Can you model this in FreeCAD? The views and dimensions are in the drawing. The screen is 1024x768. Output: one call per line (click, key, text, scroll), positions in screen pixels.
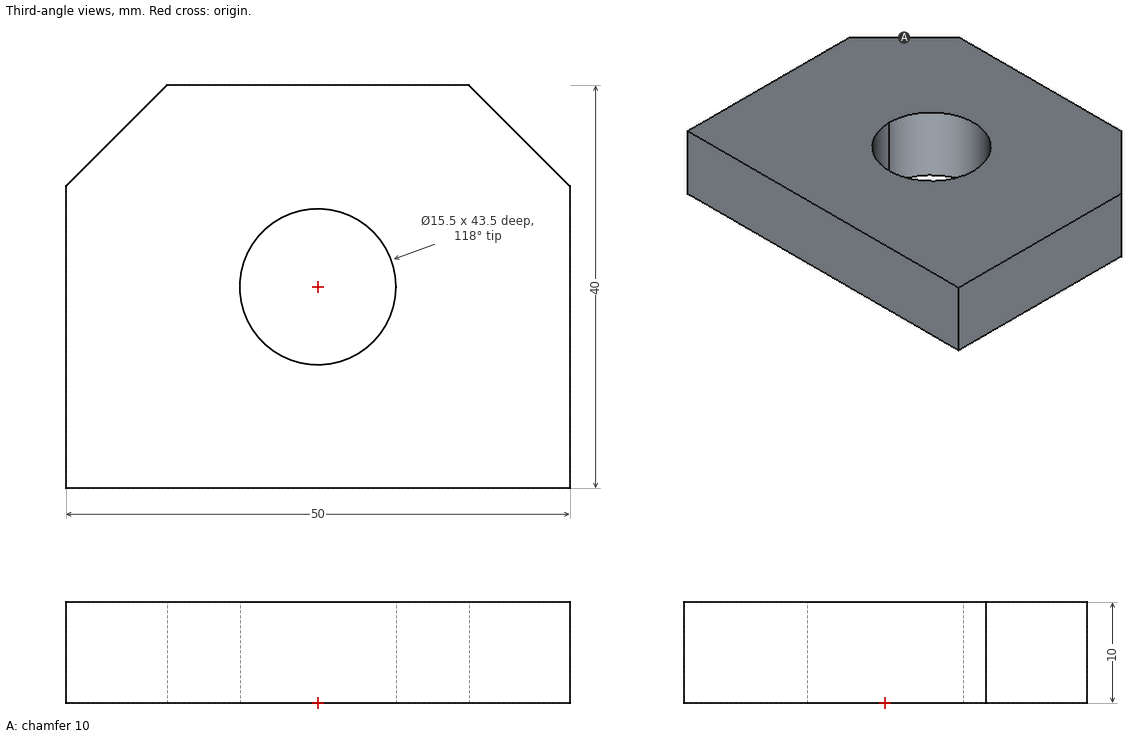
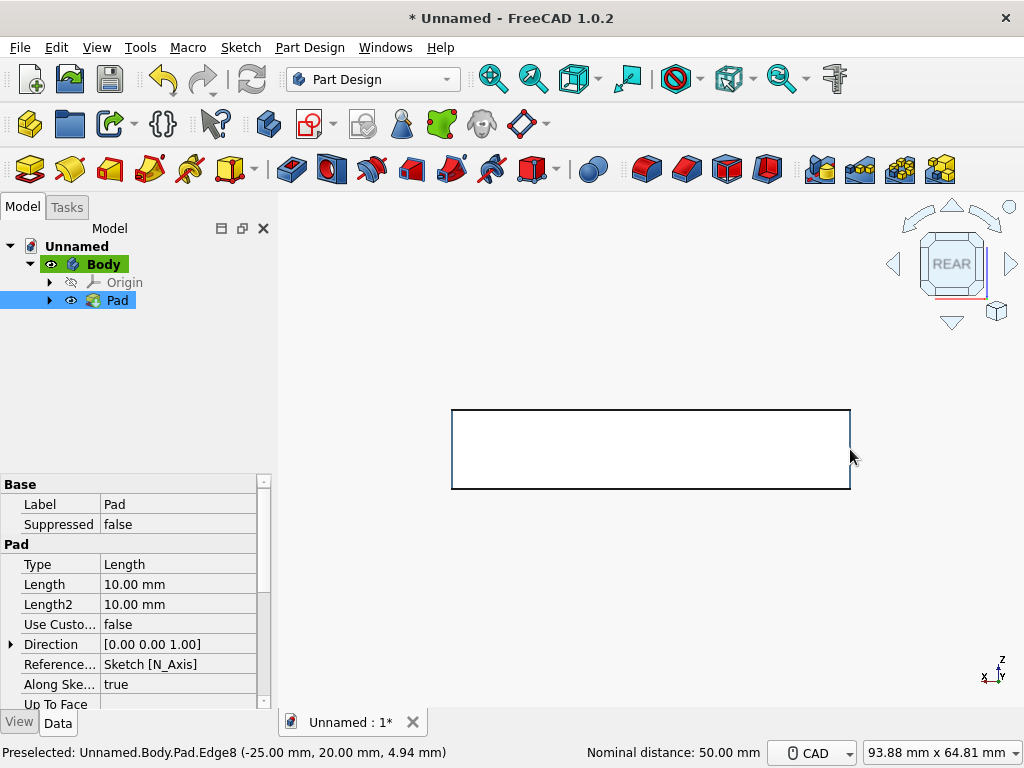
click(688, 170)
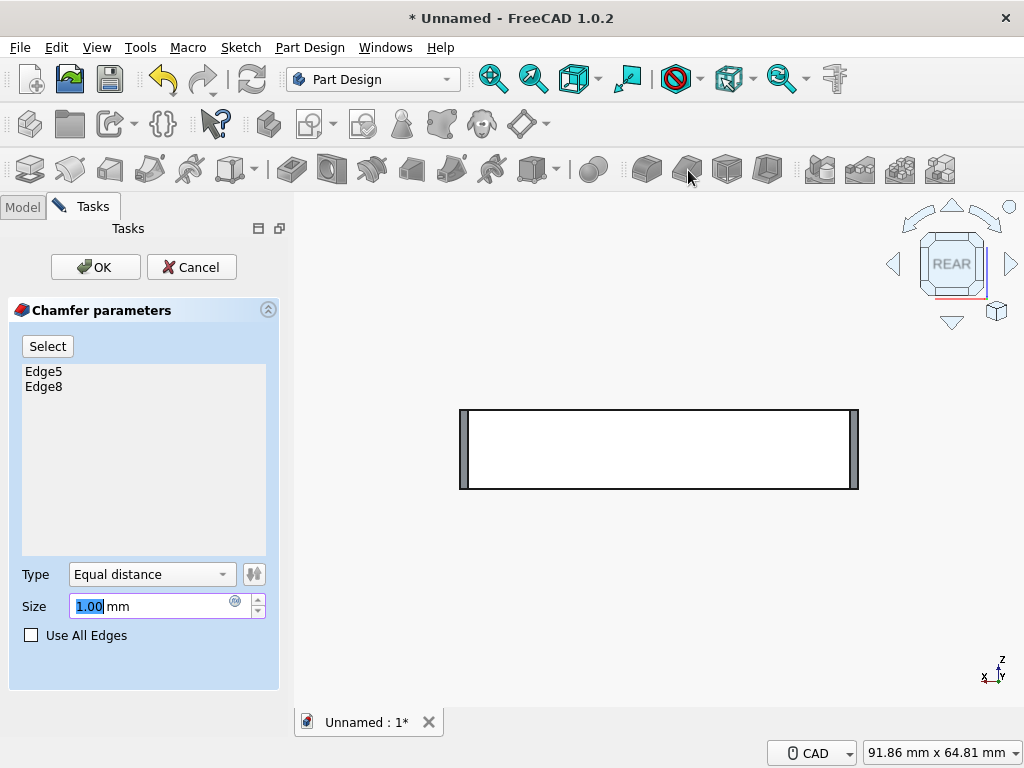
text(10)
key(Tab)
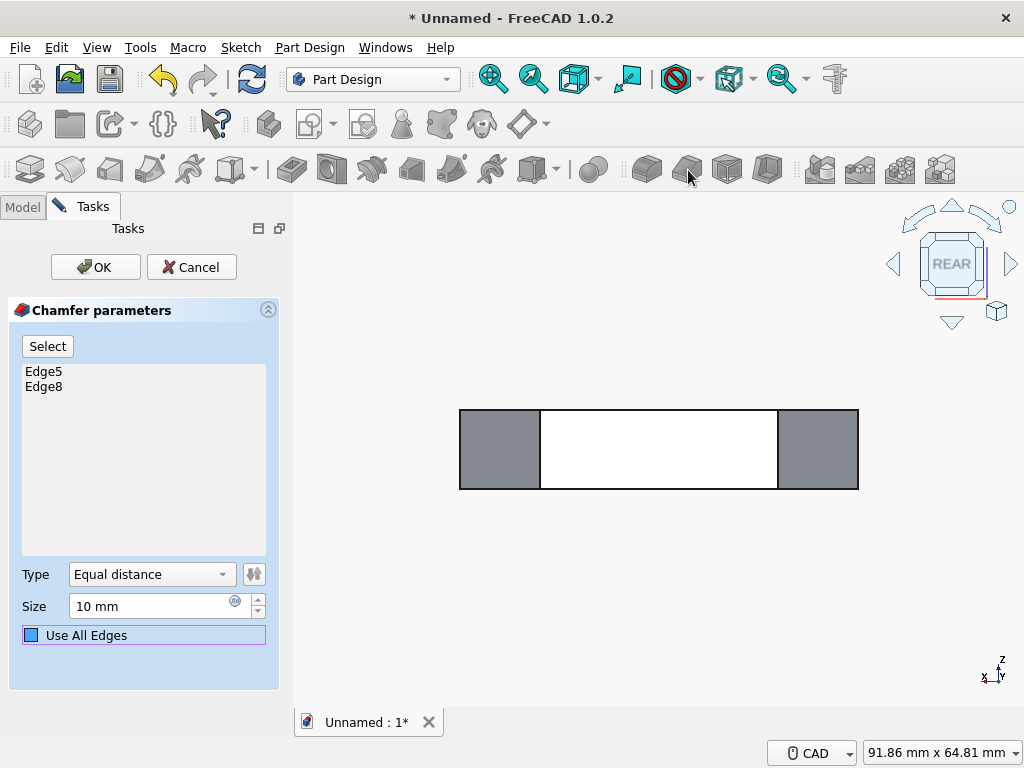
click(96, 267)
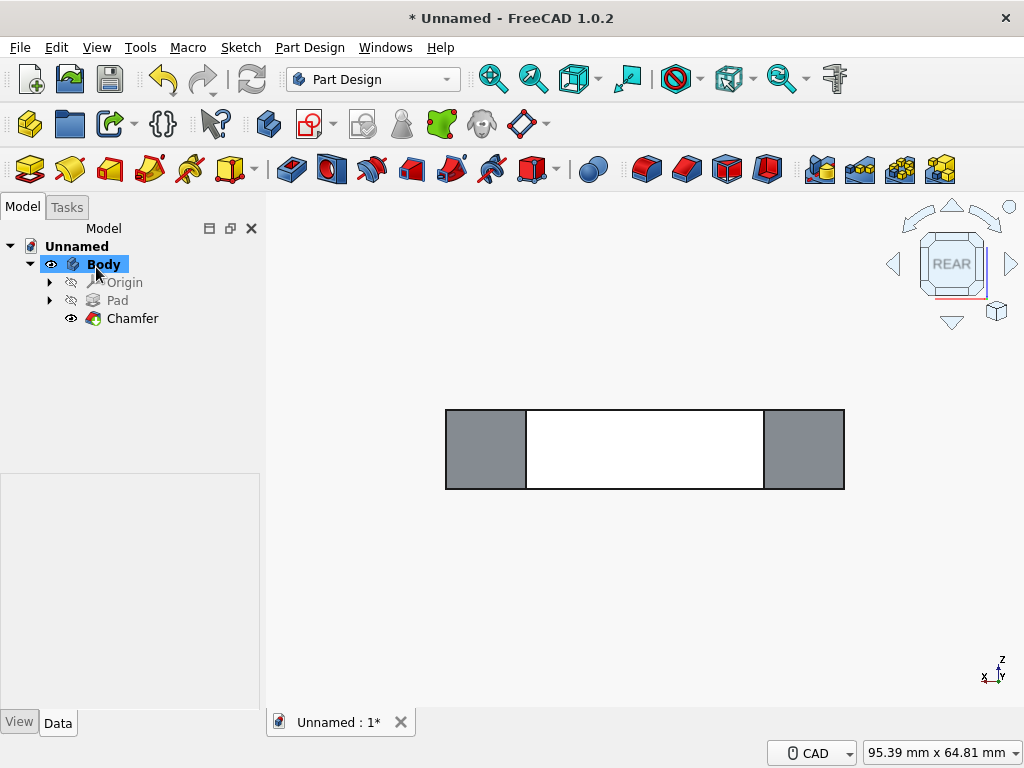
key(5)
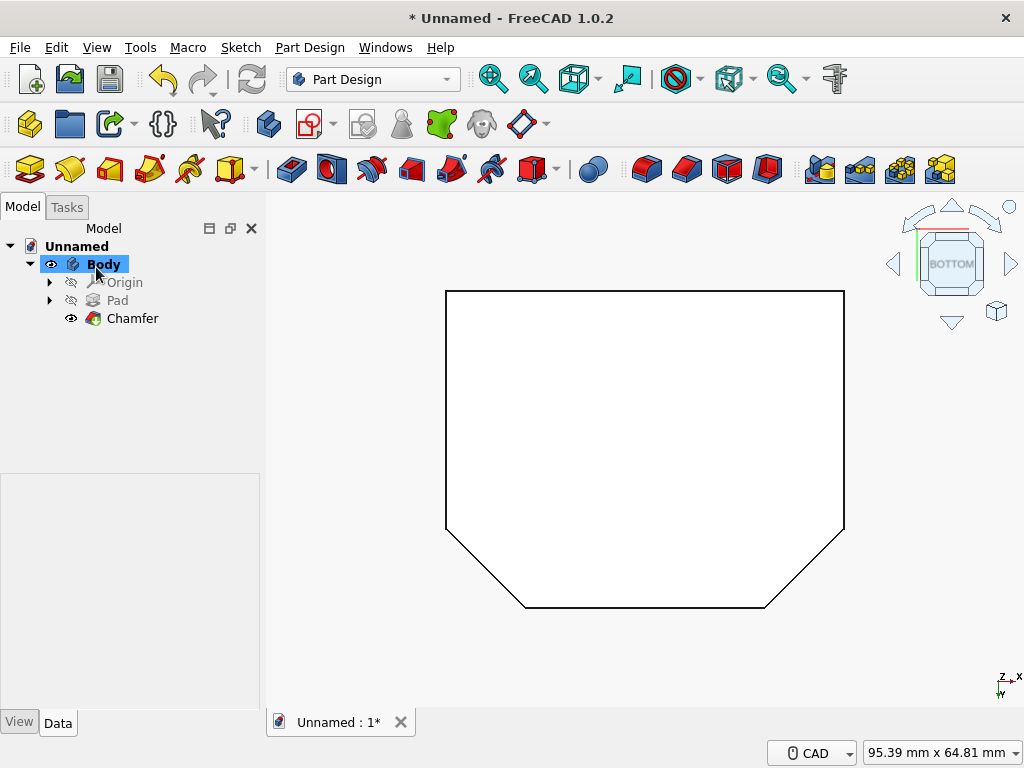
click(645, 448)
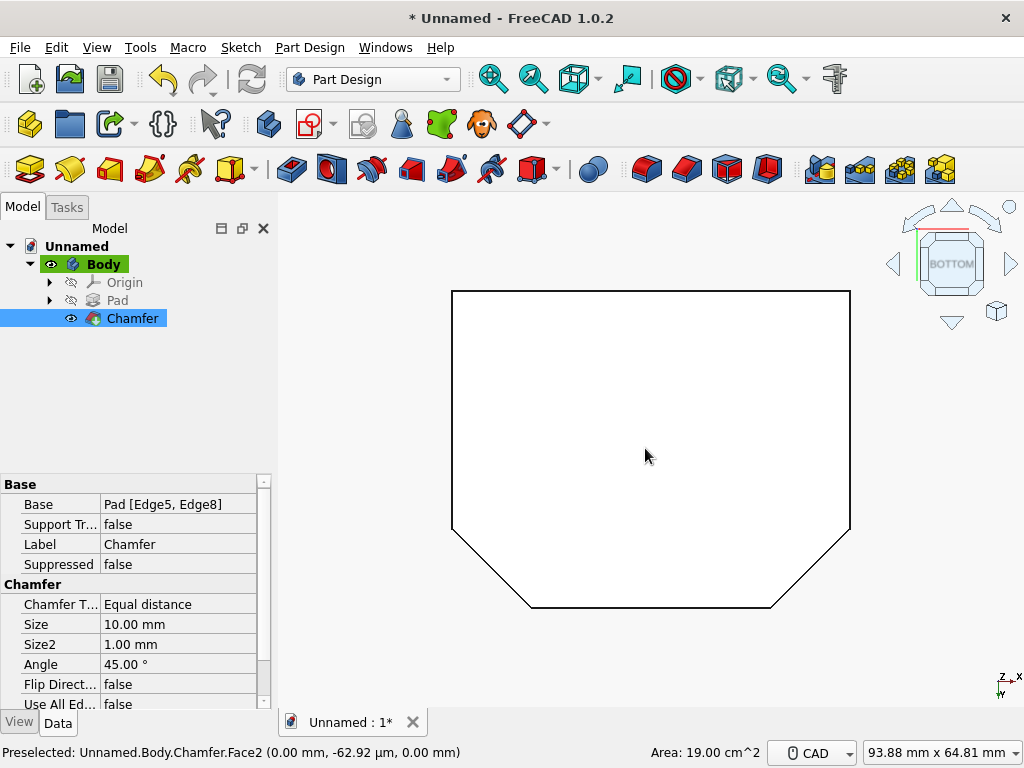
click(310, 124)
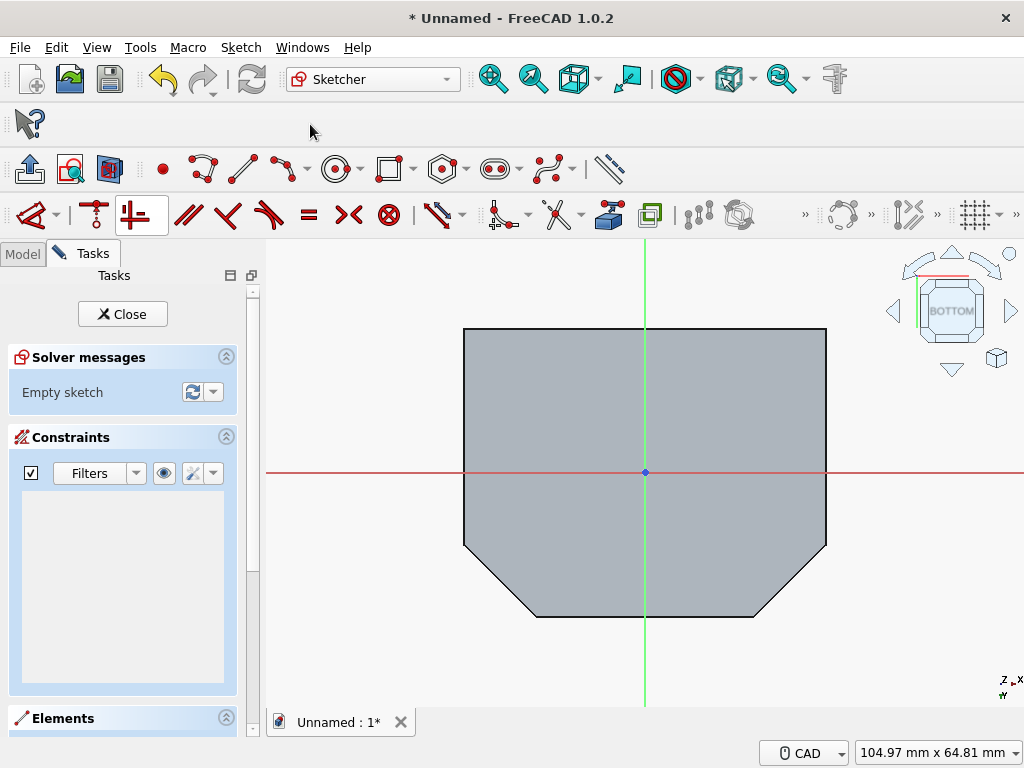
scroll(685, 473, up, 5)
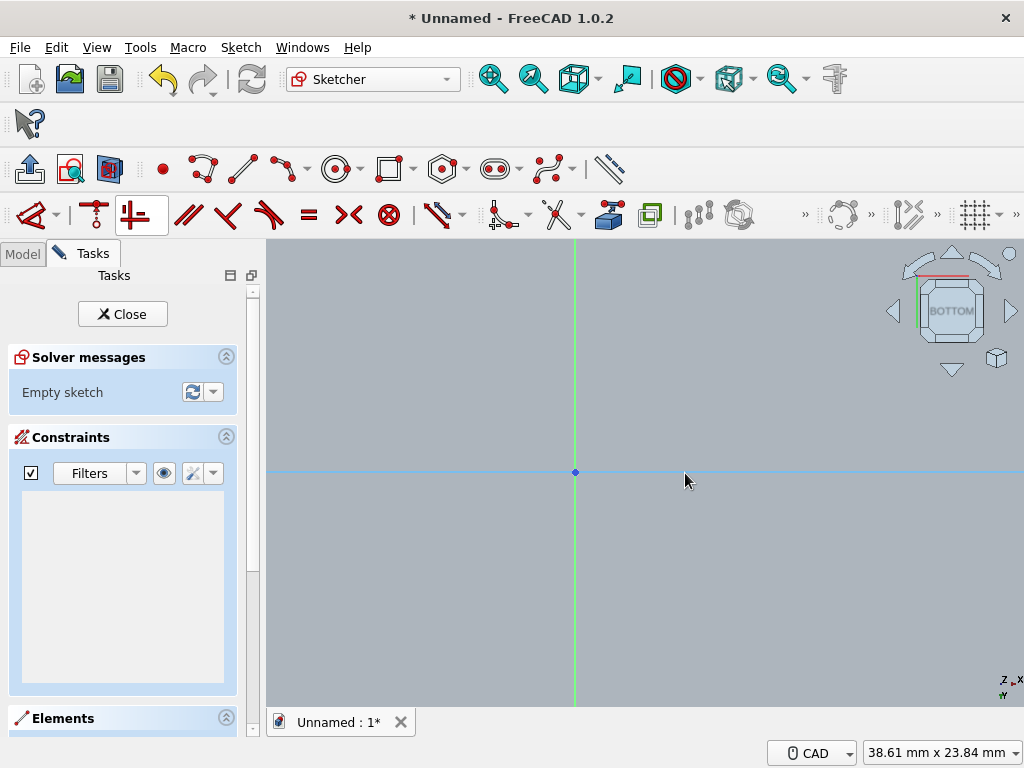
key(g)
key(c)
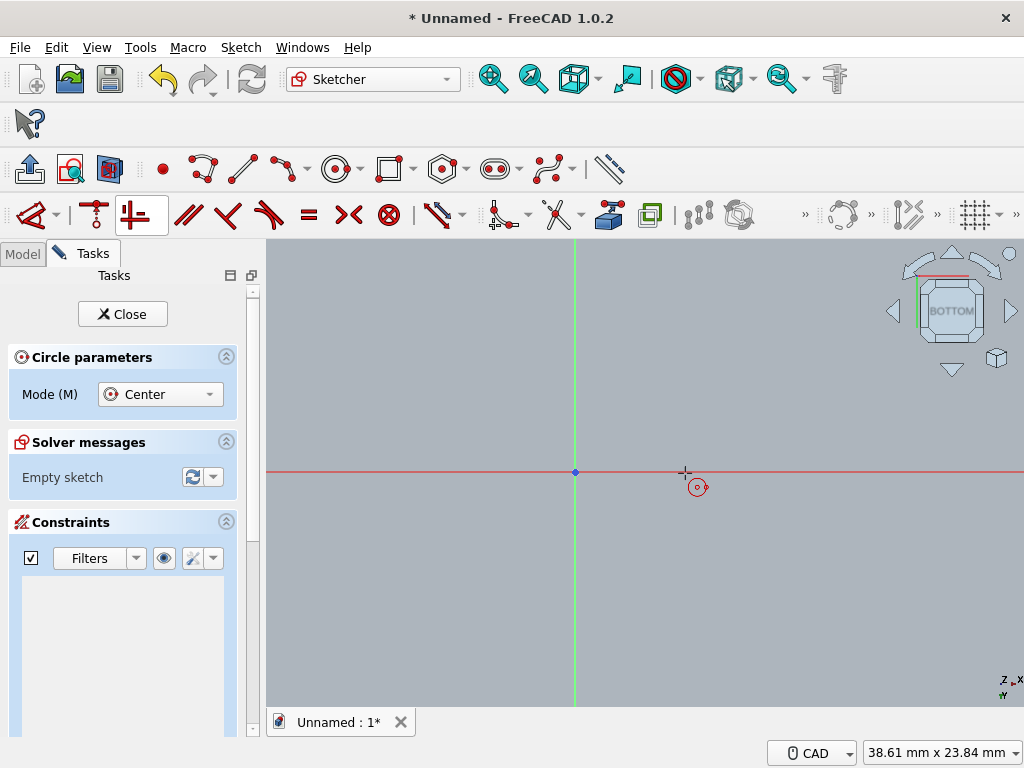
click(575, 472)
click(683, 365)
key(Escape)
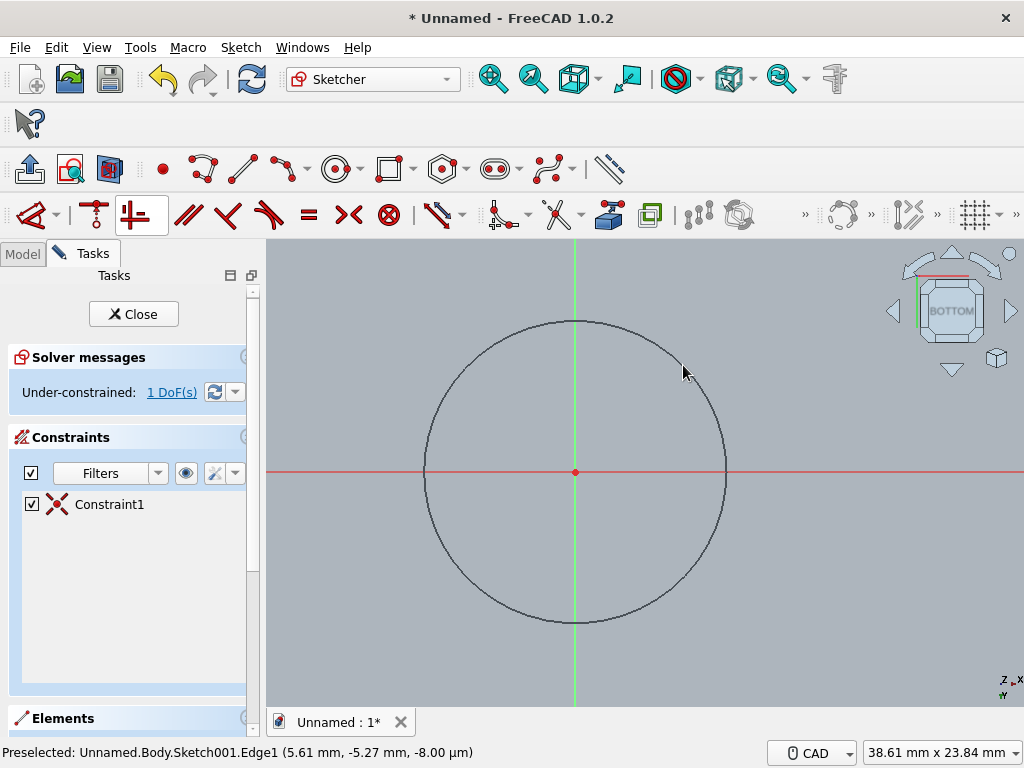
click(32, 216)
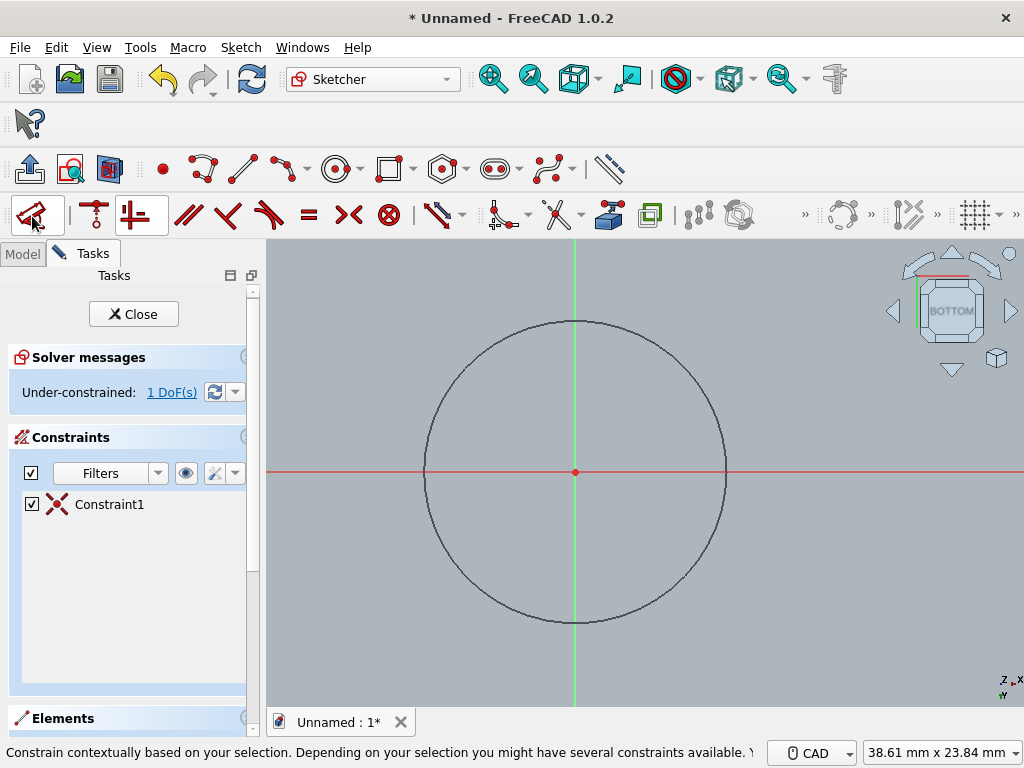
click(682, 365)
click(705, 342)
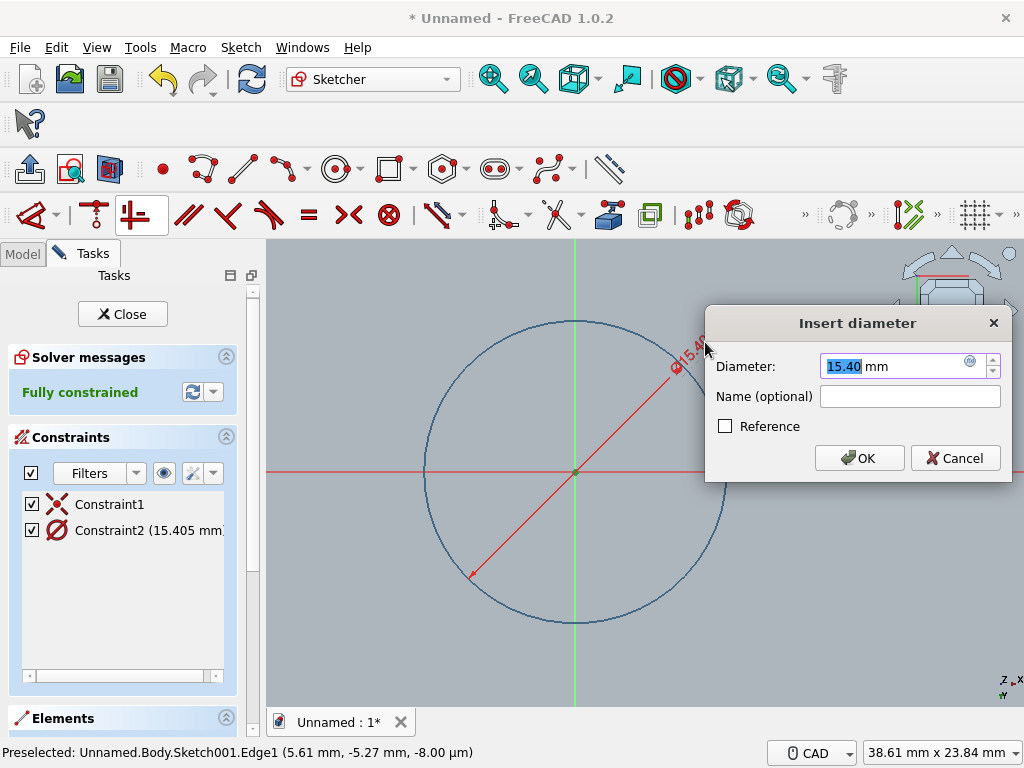
text(15.5)
key(Return)
key(Escape)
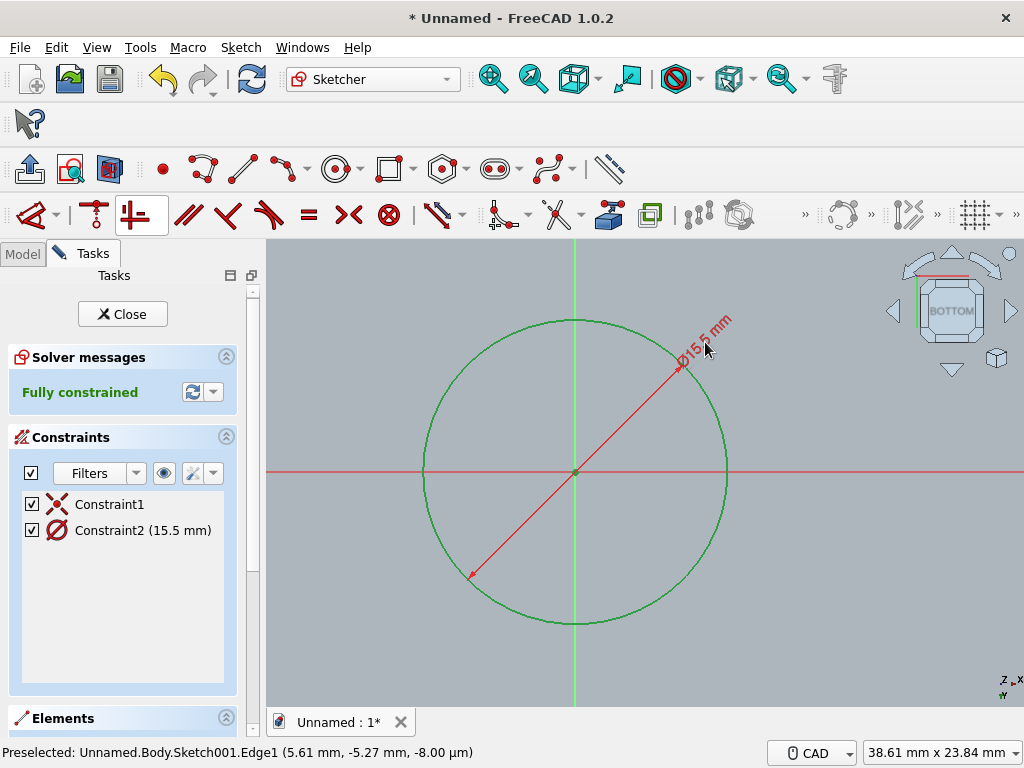
click(123, 314)